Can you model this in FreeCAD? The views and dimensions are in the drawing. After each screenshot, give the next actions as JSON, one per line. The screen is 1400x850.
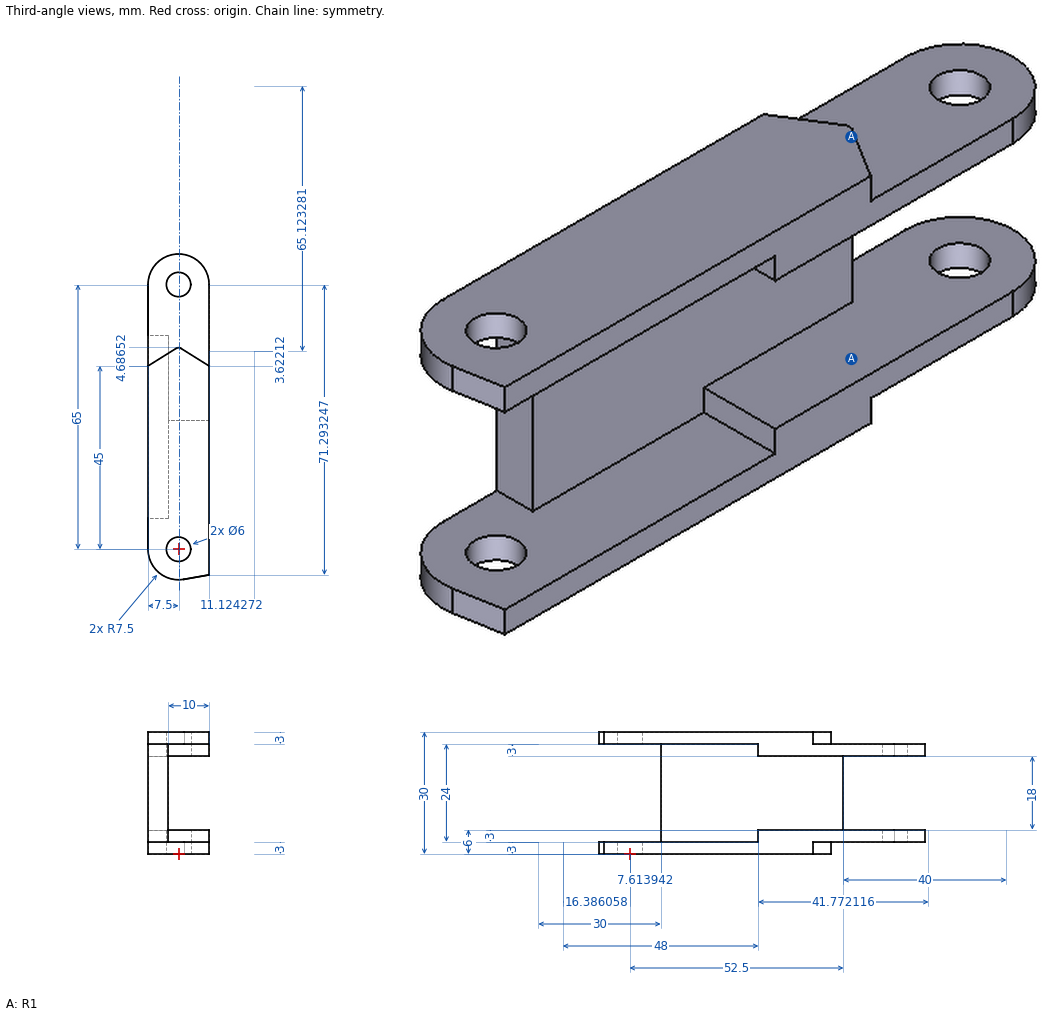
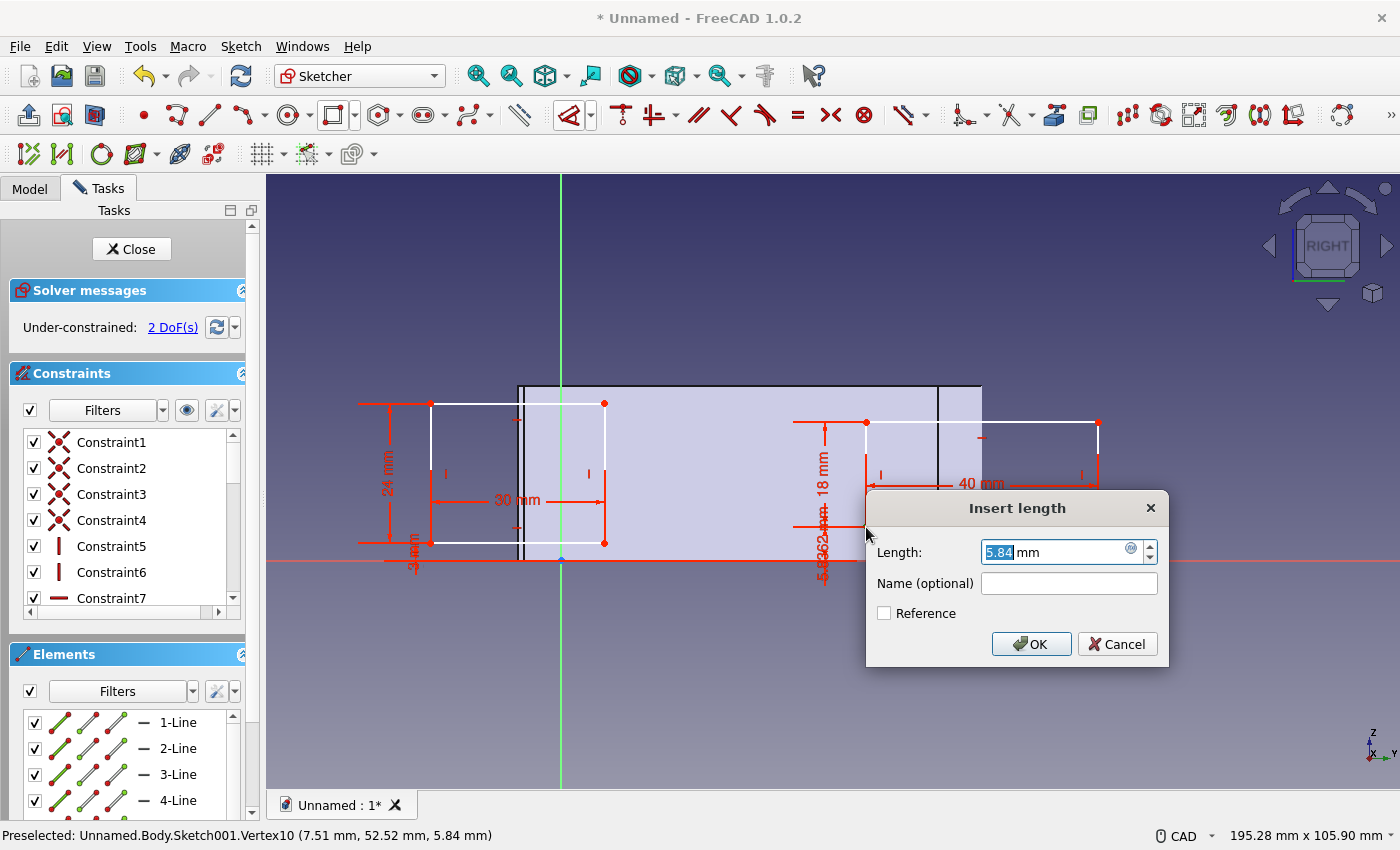
{"action": "type", "text": "6"}
{"action": "key", "text": "Return"}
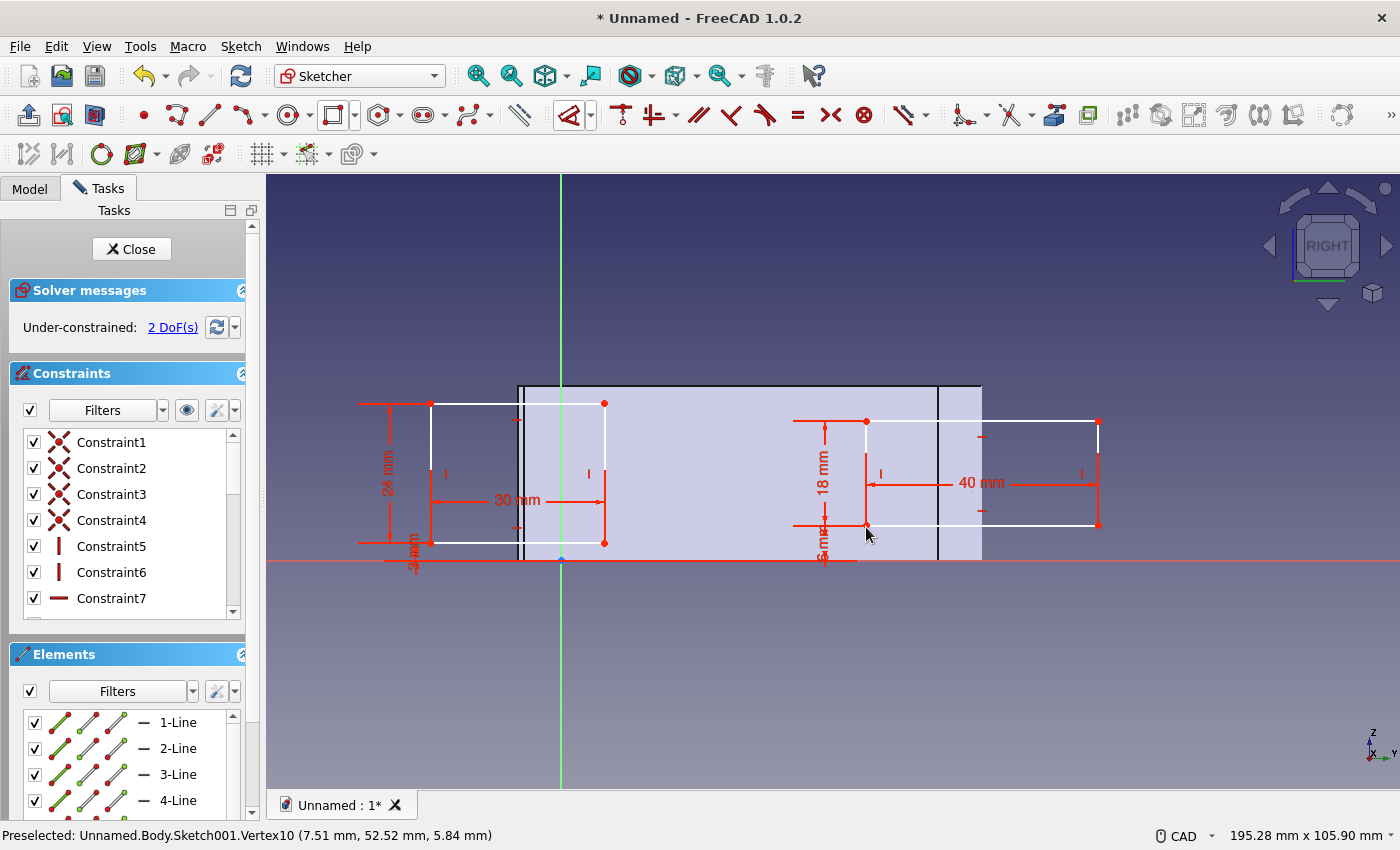
{"action": "left_click", "coordinate": [866, 421]}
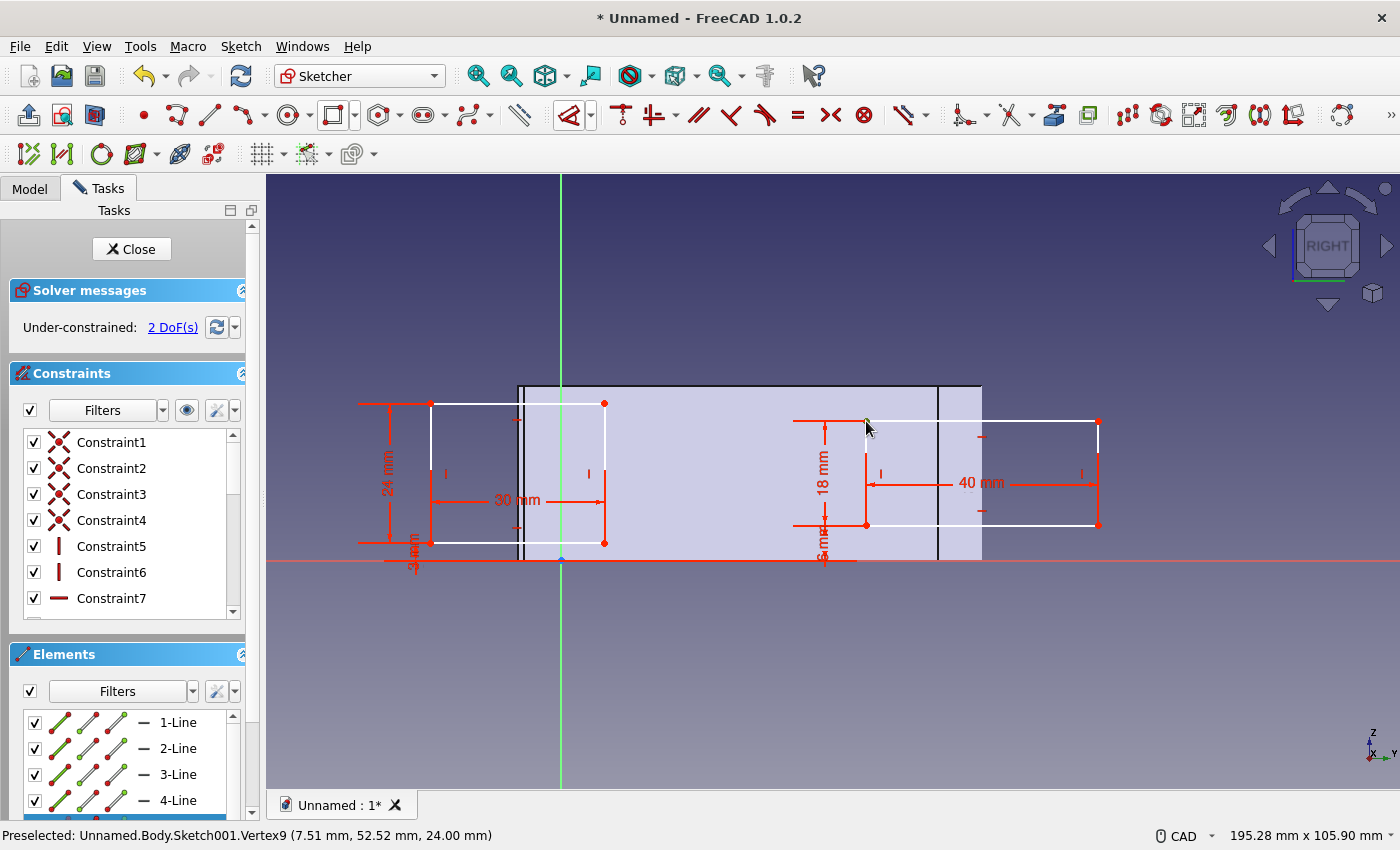
{"action": "key", "text": "l"}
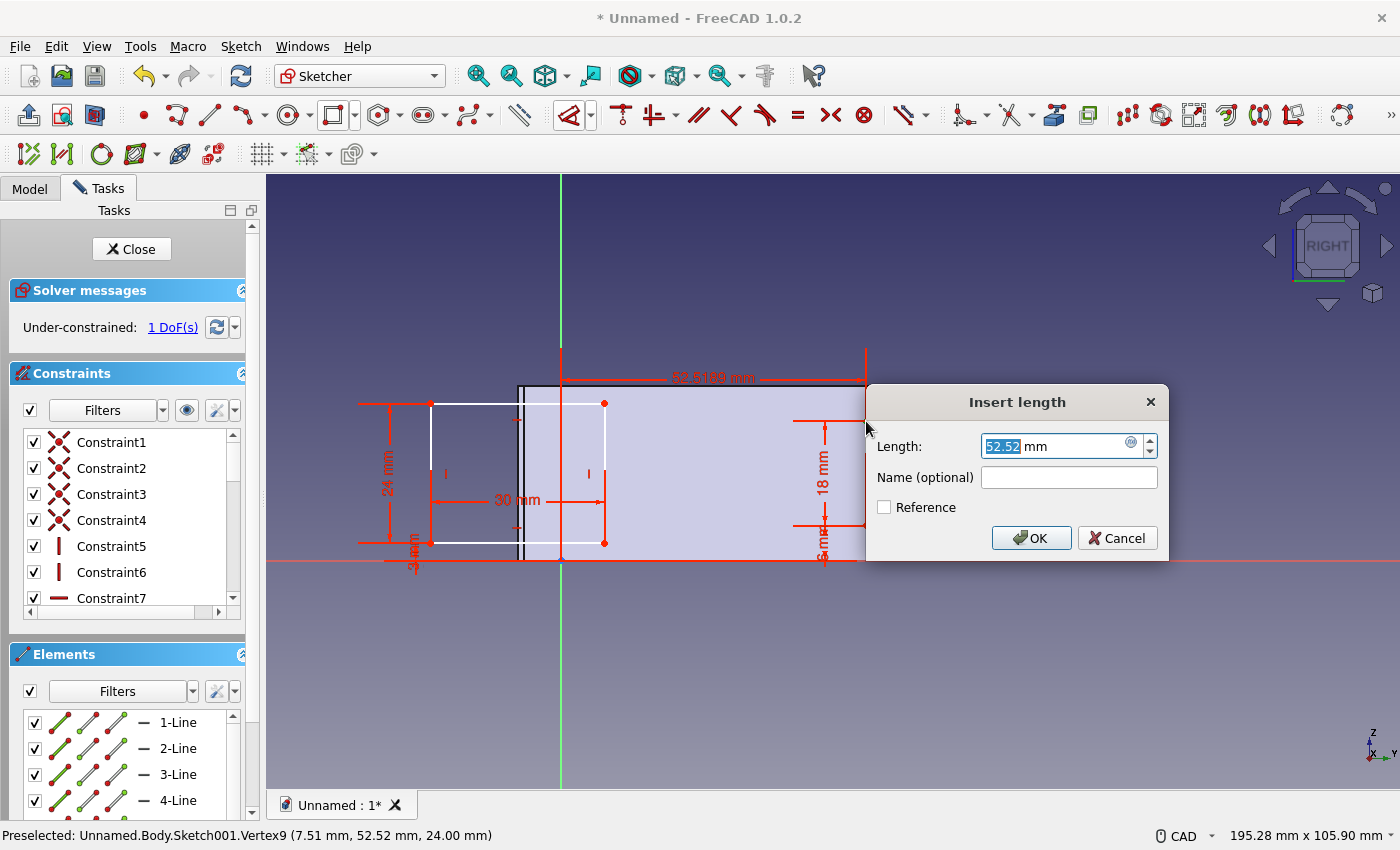
{"action": "type", "text": "52.5"}
{"action": "key", "text": "Return"}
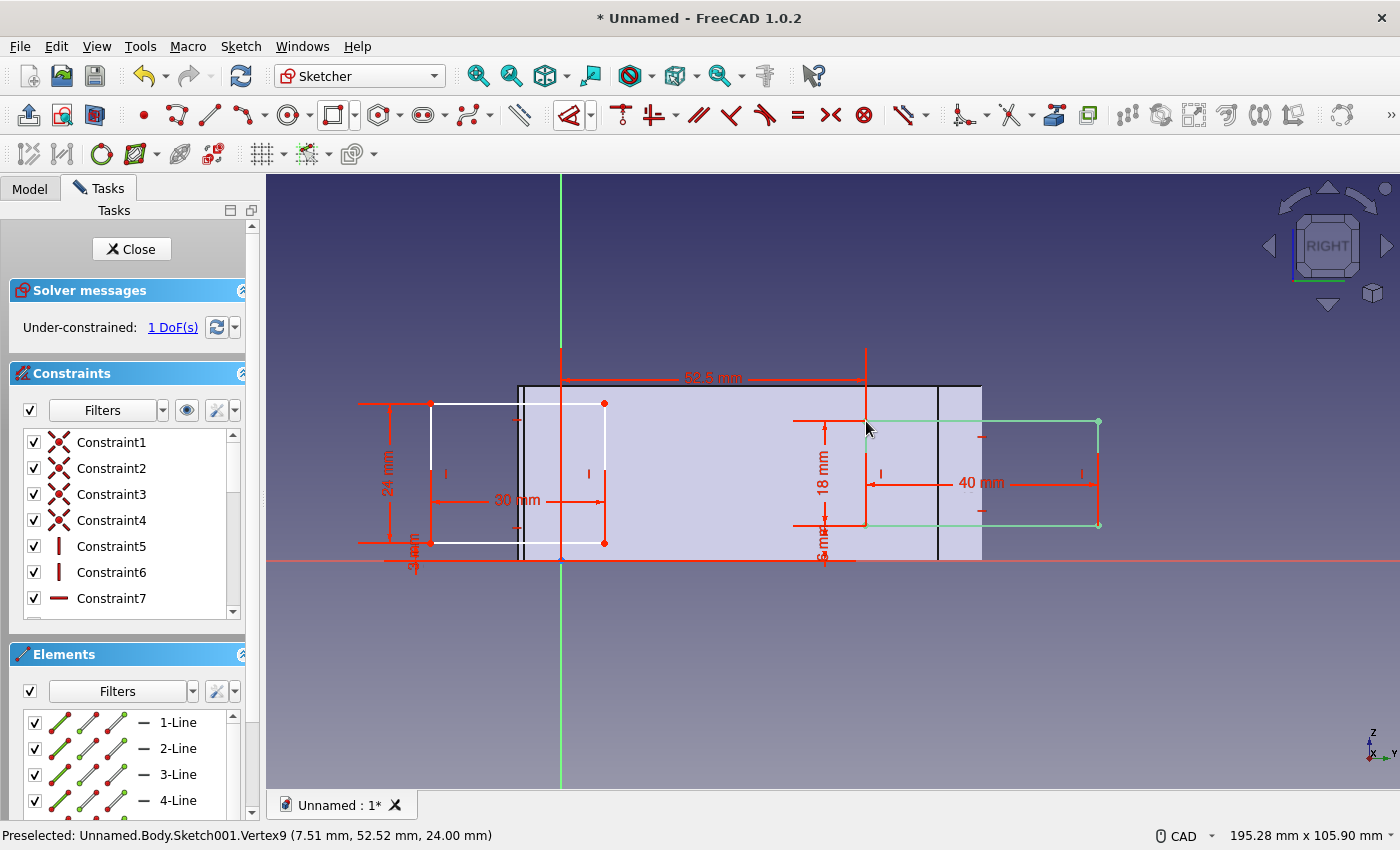
{"action": "left_click", "coordinate": [605, 543]}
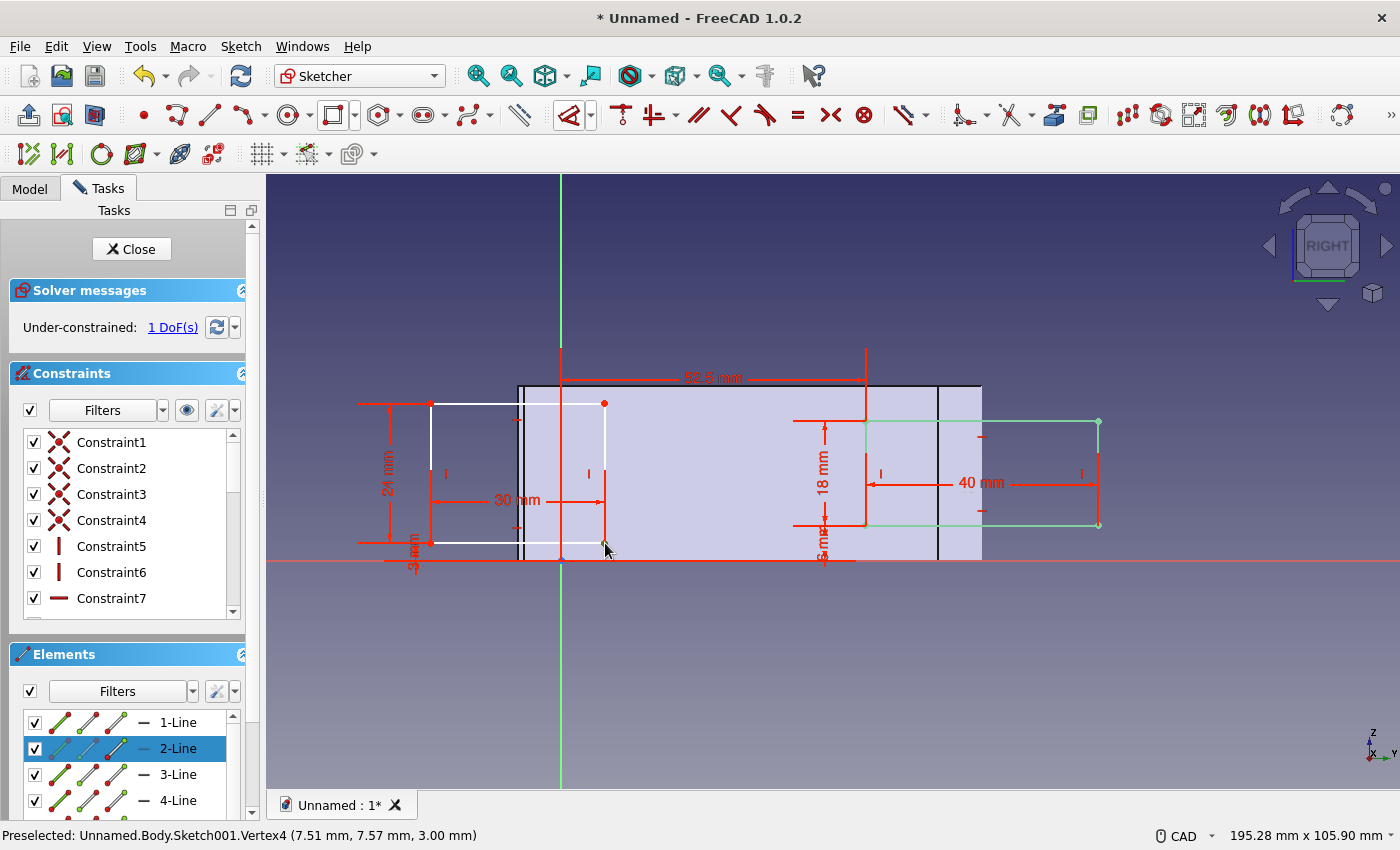
{"action": "key", "text": "l"}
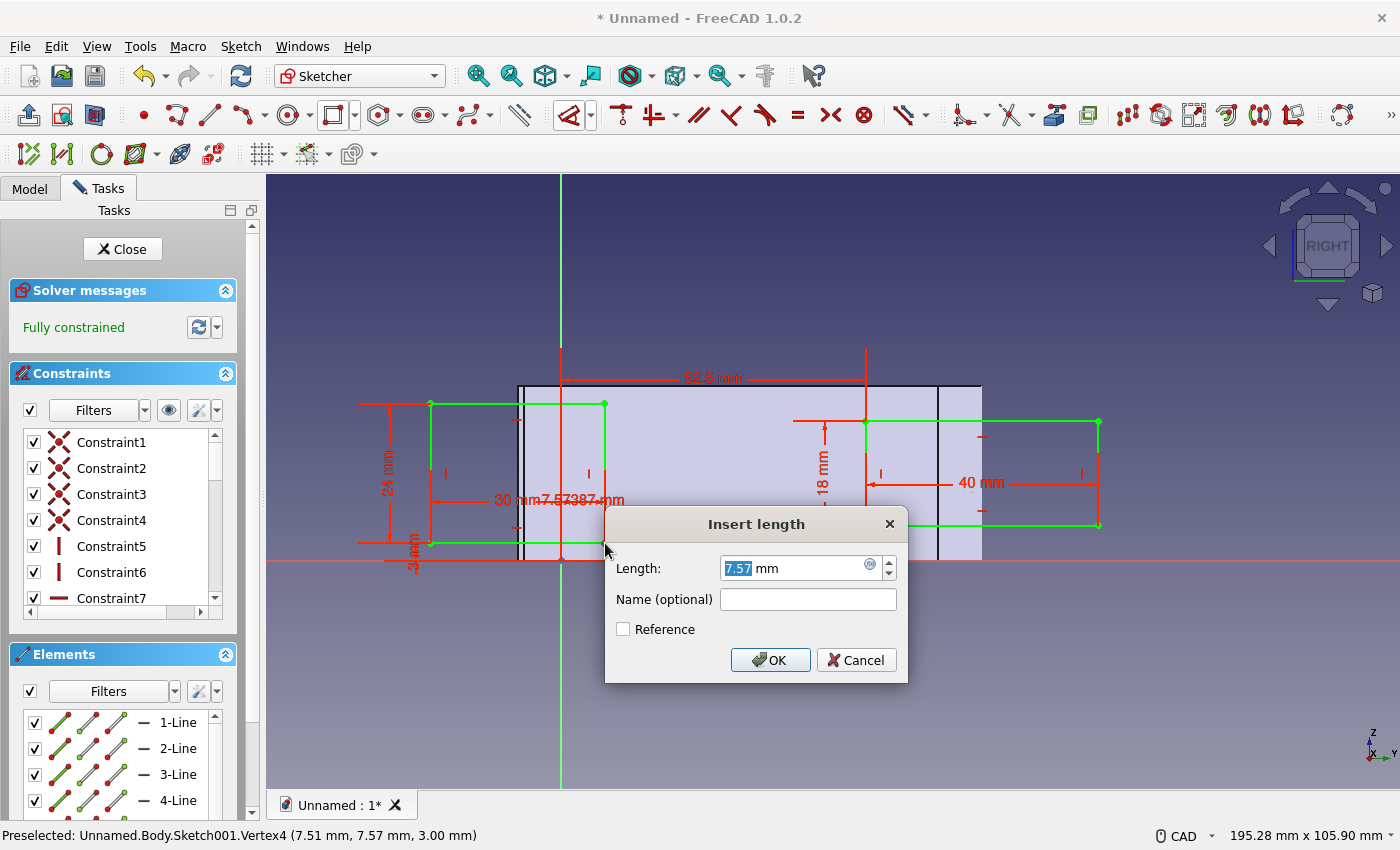
{"action": "type", "text": "7.613942"}
{"action": "key", "text": "Return"}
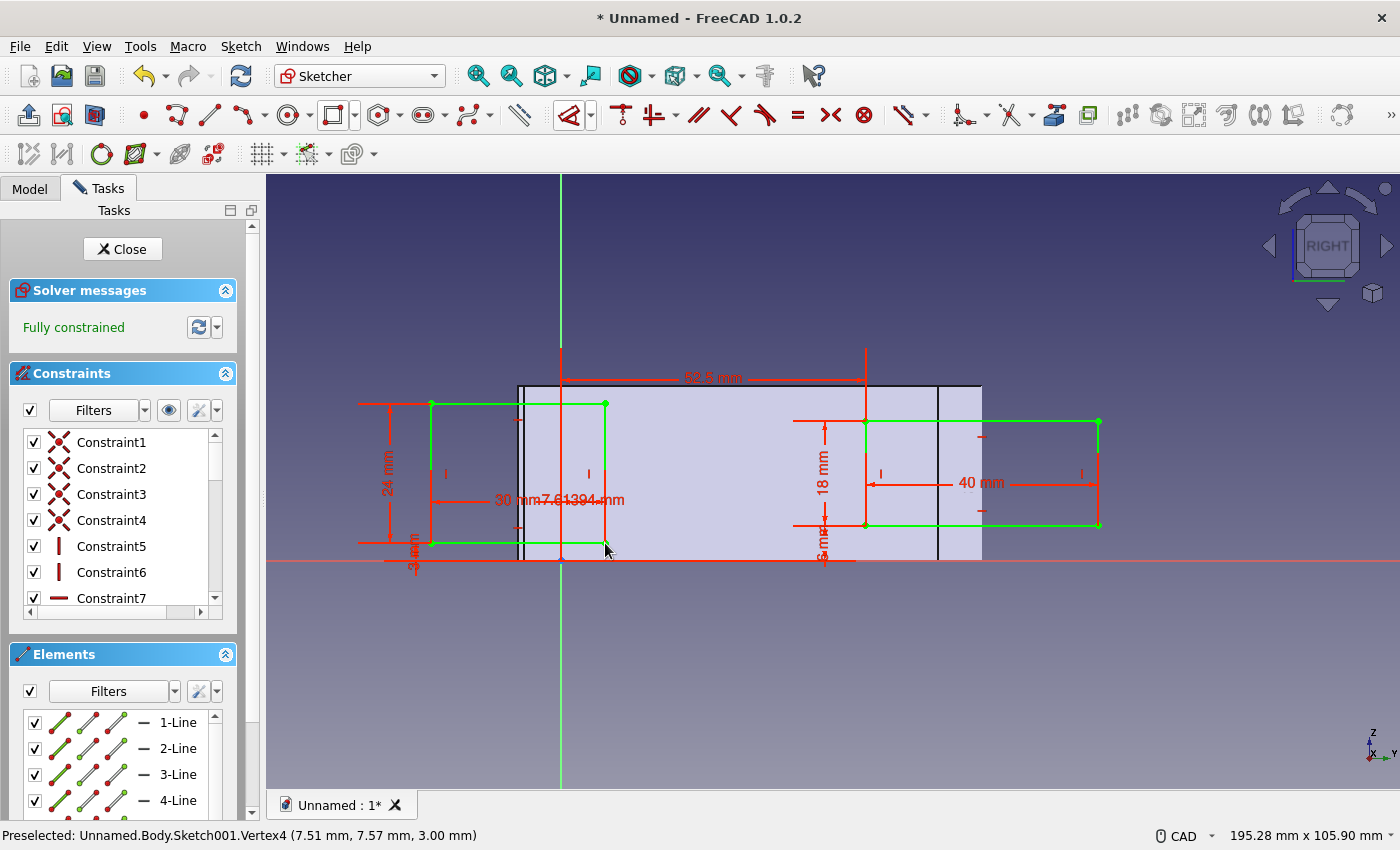
{"action": "left_click", "coordinate": [123, 249]}